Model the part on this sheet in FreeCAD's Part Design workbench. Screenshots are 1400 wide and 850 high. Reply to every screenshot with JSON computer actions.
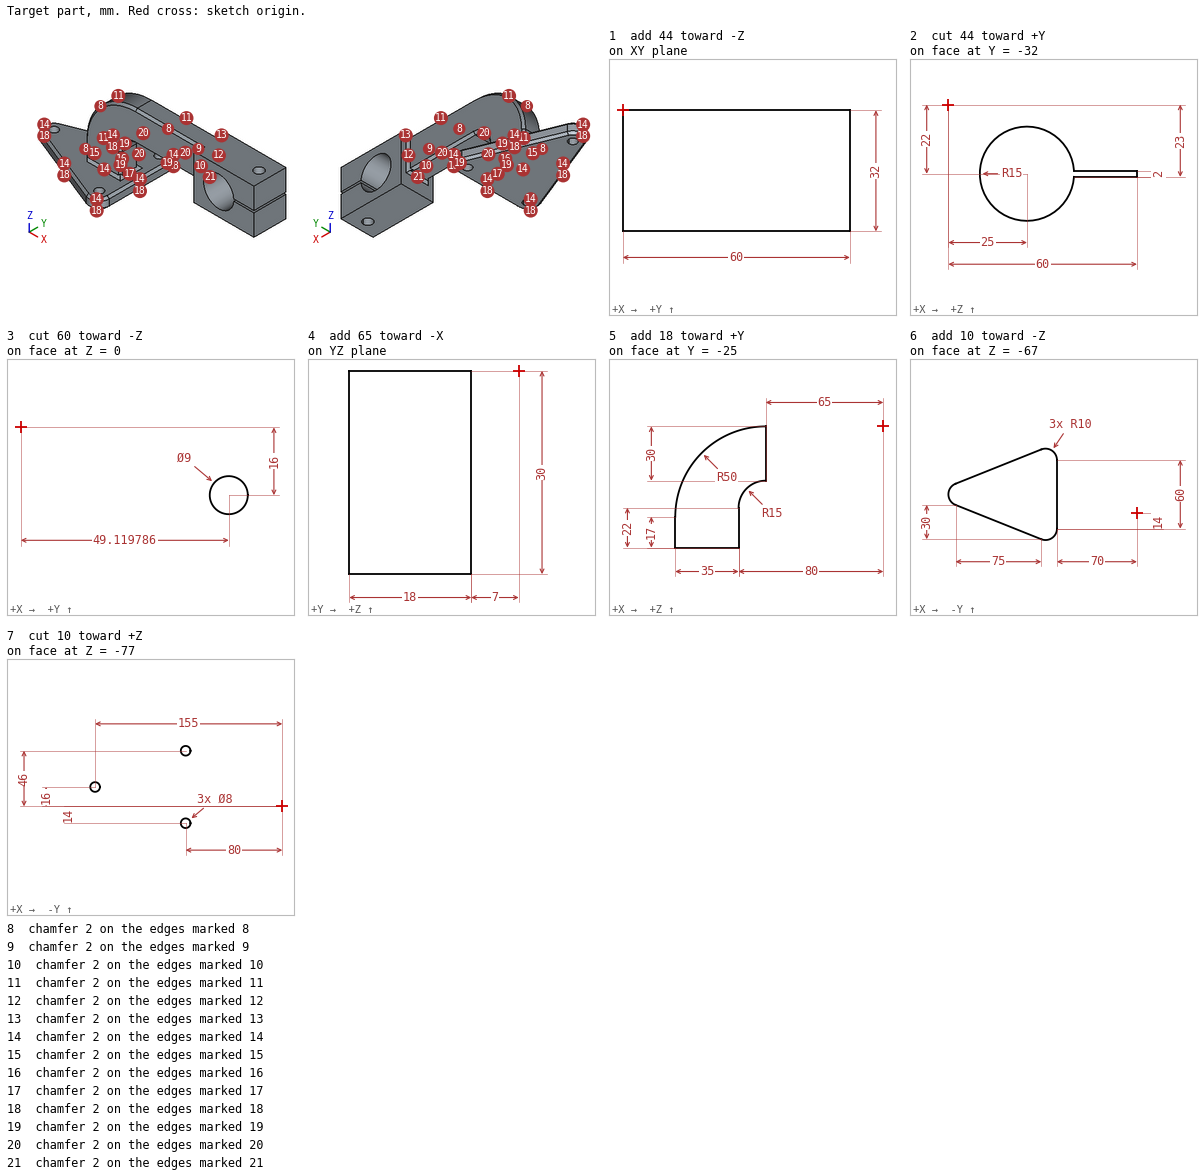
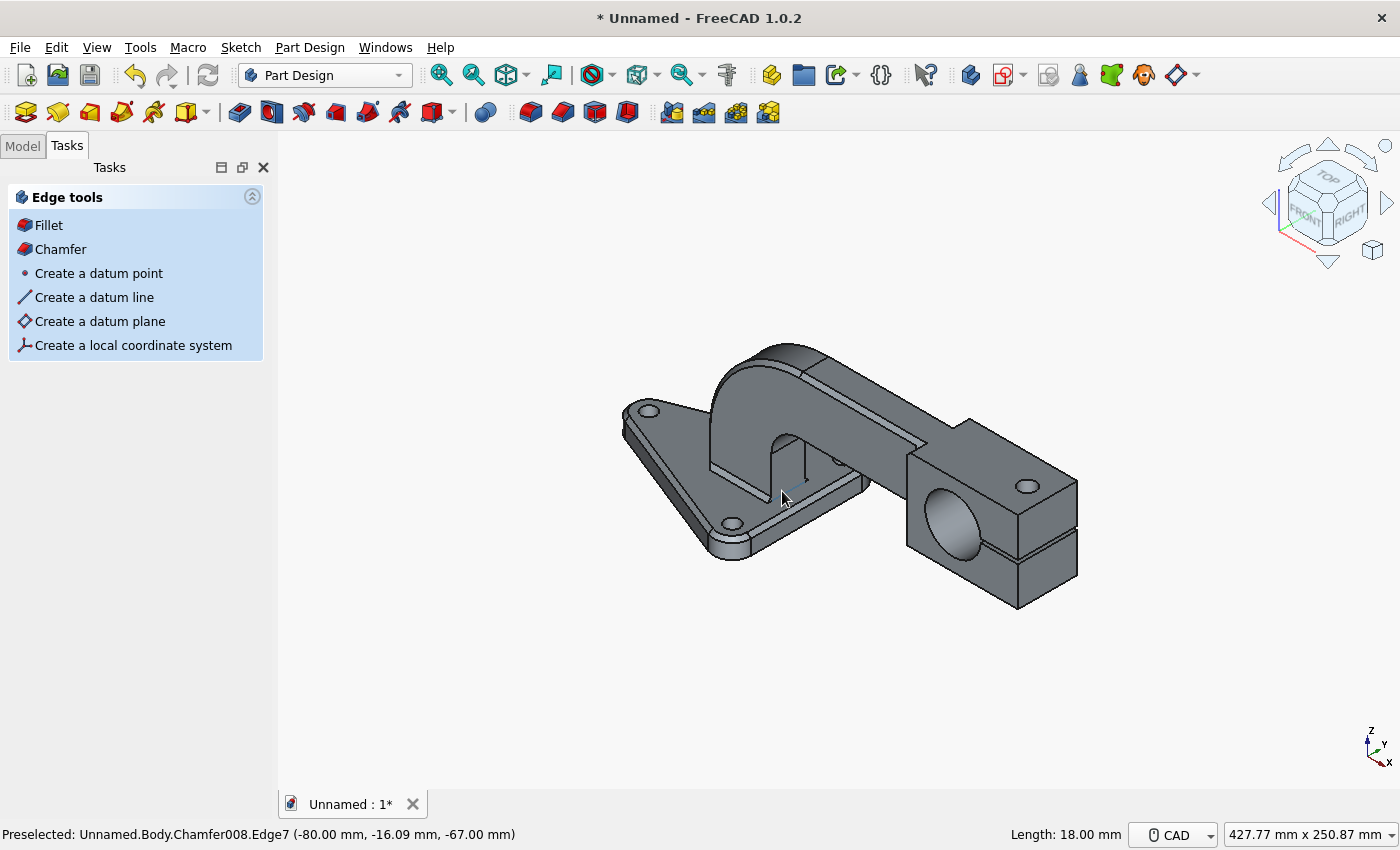
{"action": "left_click", "coordinate": [564, 112]}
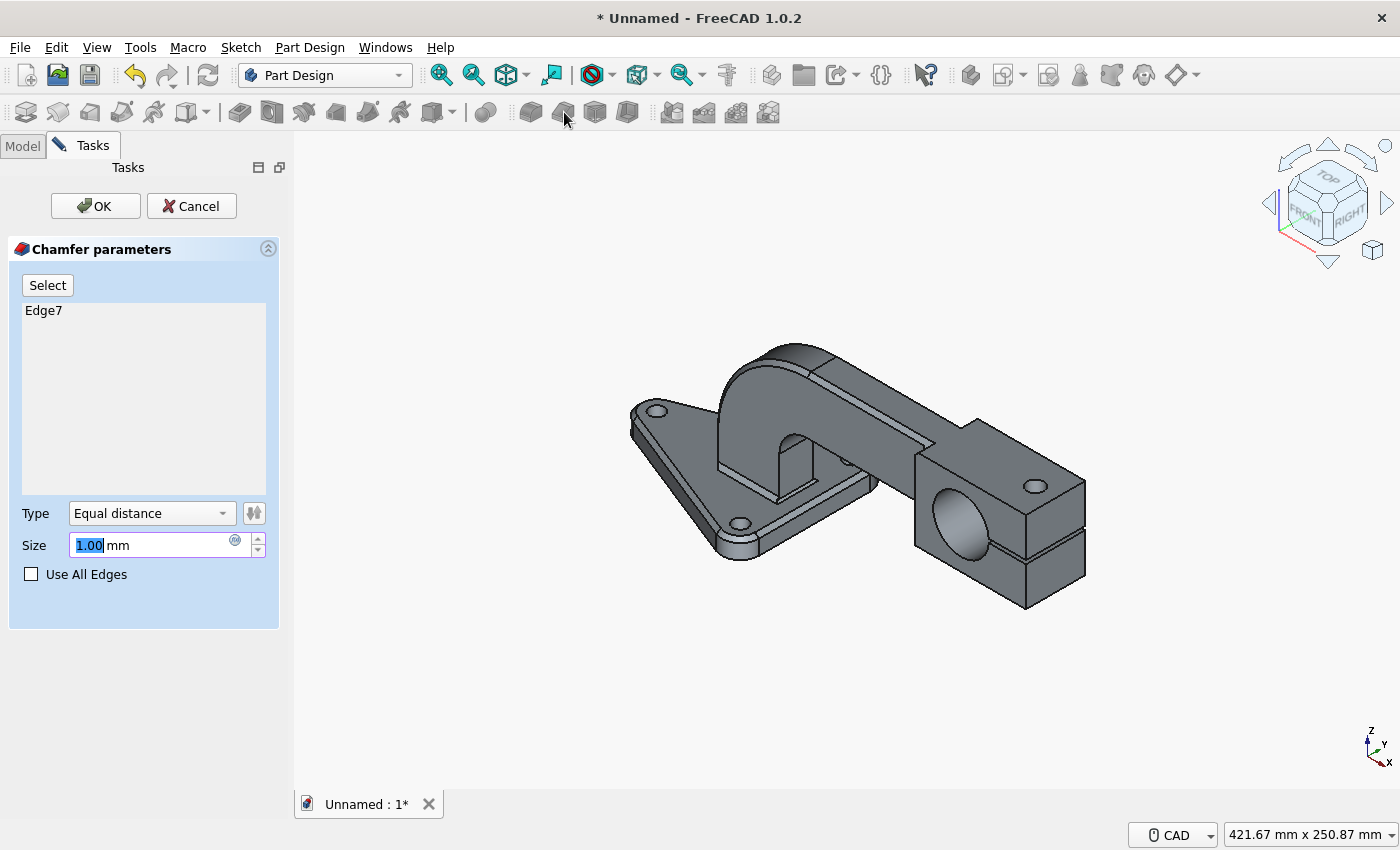
{"action": "type", "text": "2"}
{"action": "key", "text": "Tab"}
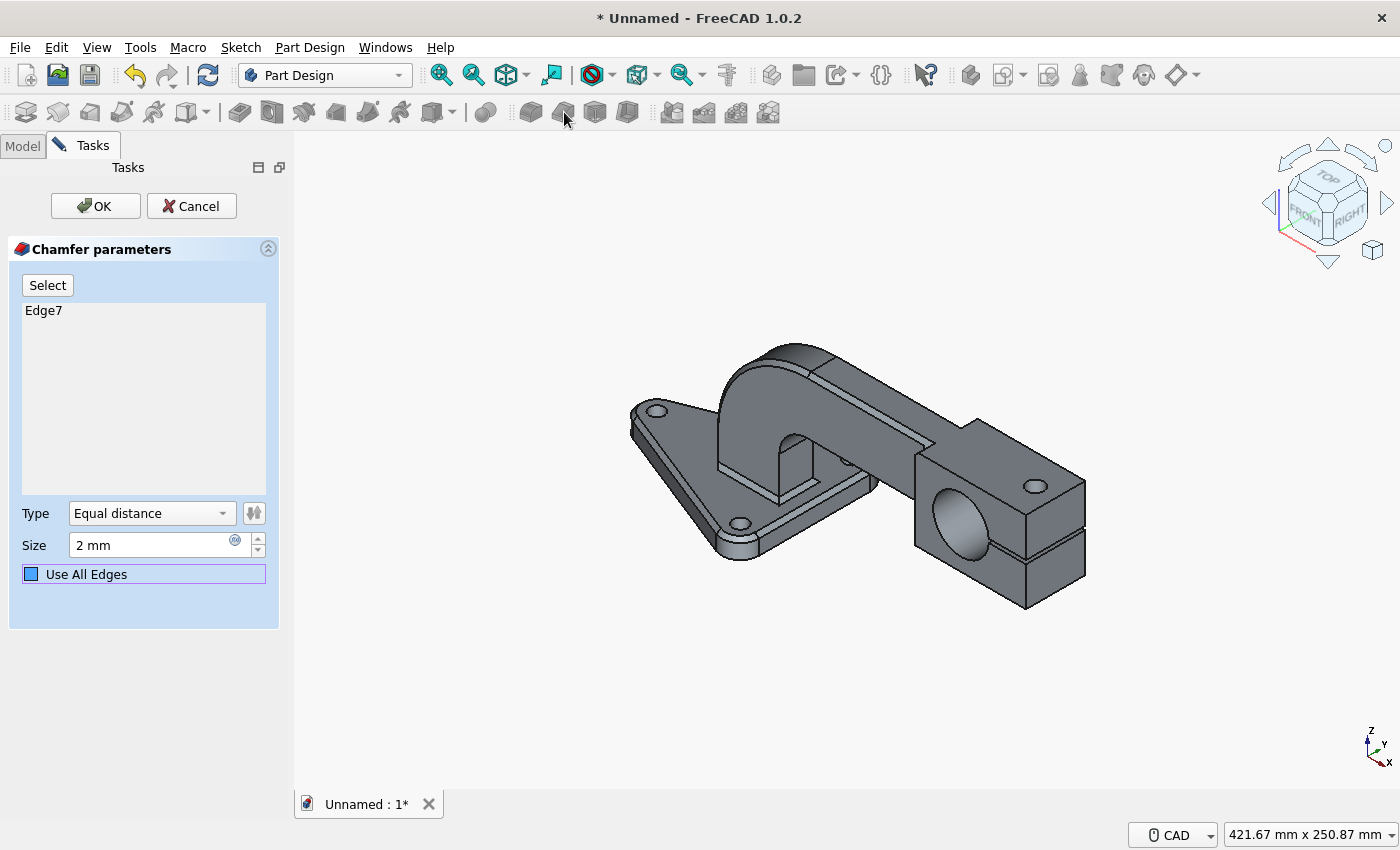
{"action": "left_click", "coordinate": [96, 206]}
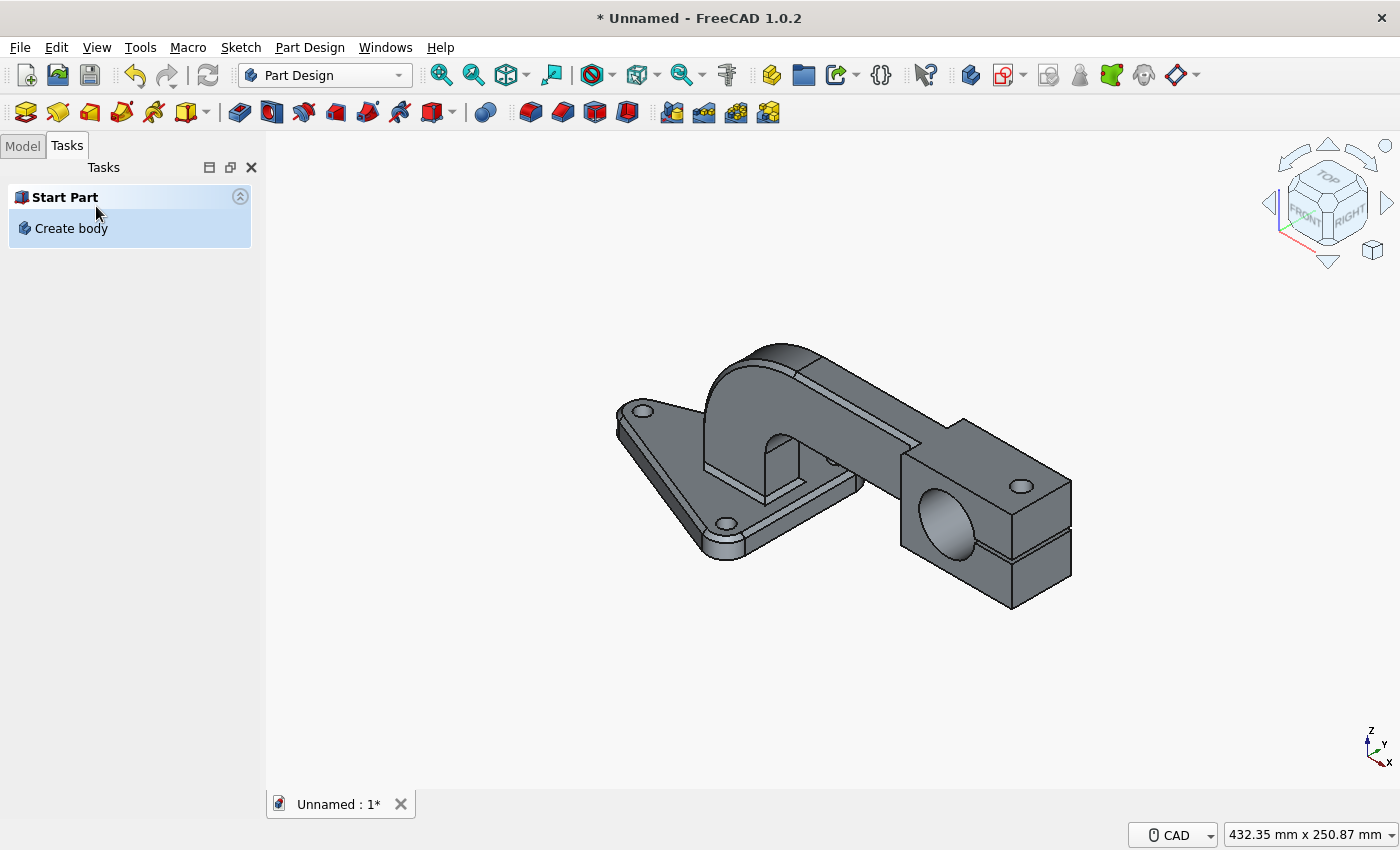
{"action": "left_click", "coordinate": [712, 557]}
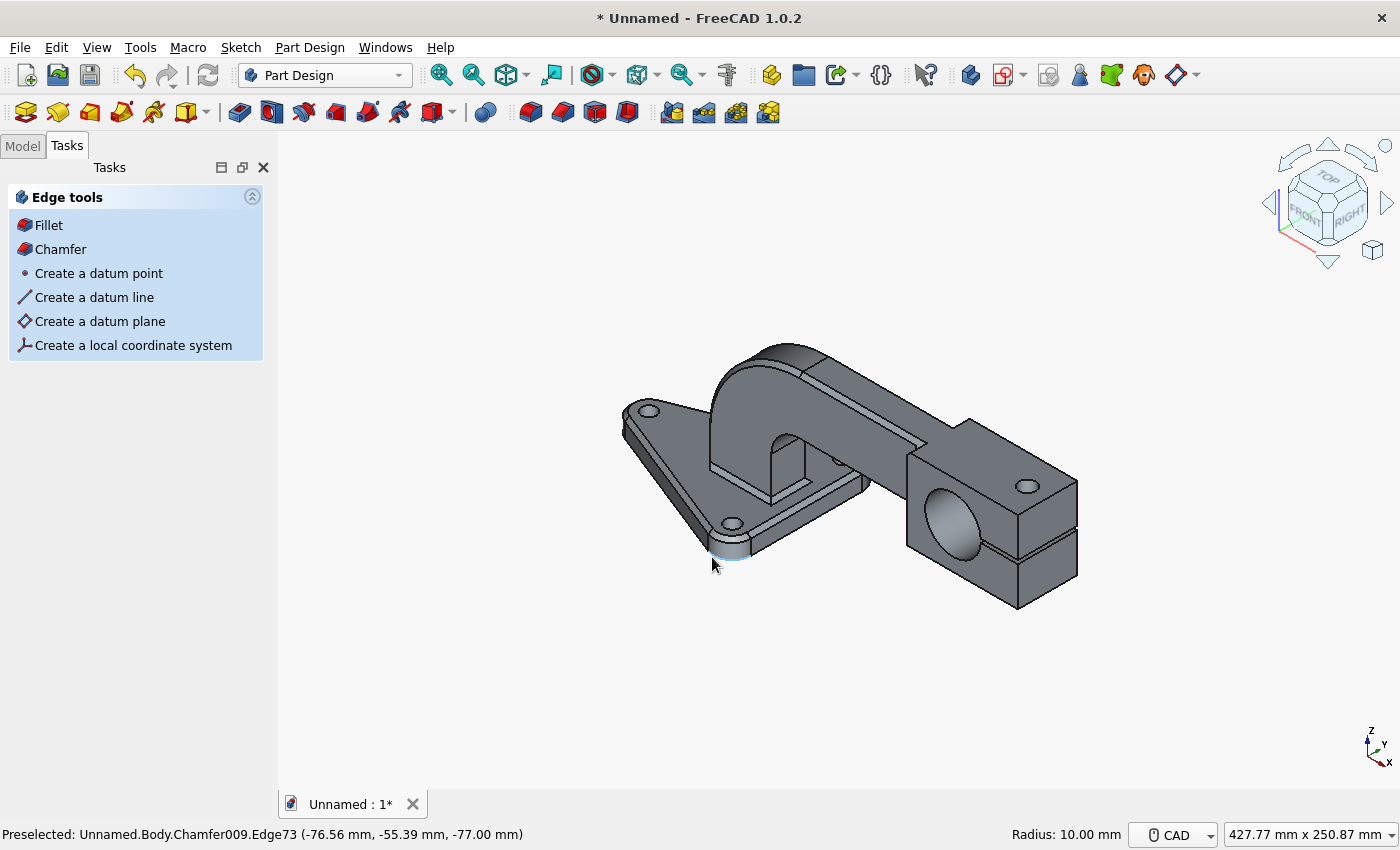
{"action": "key", "text": "2"}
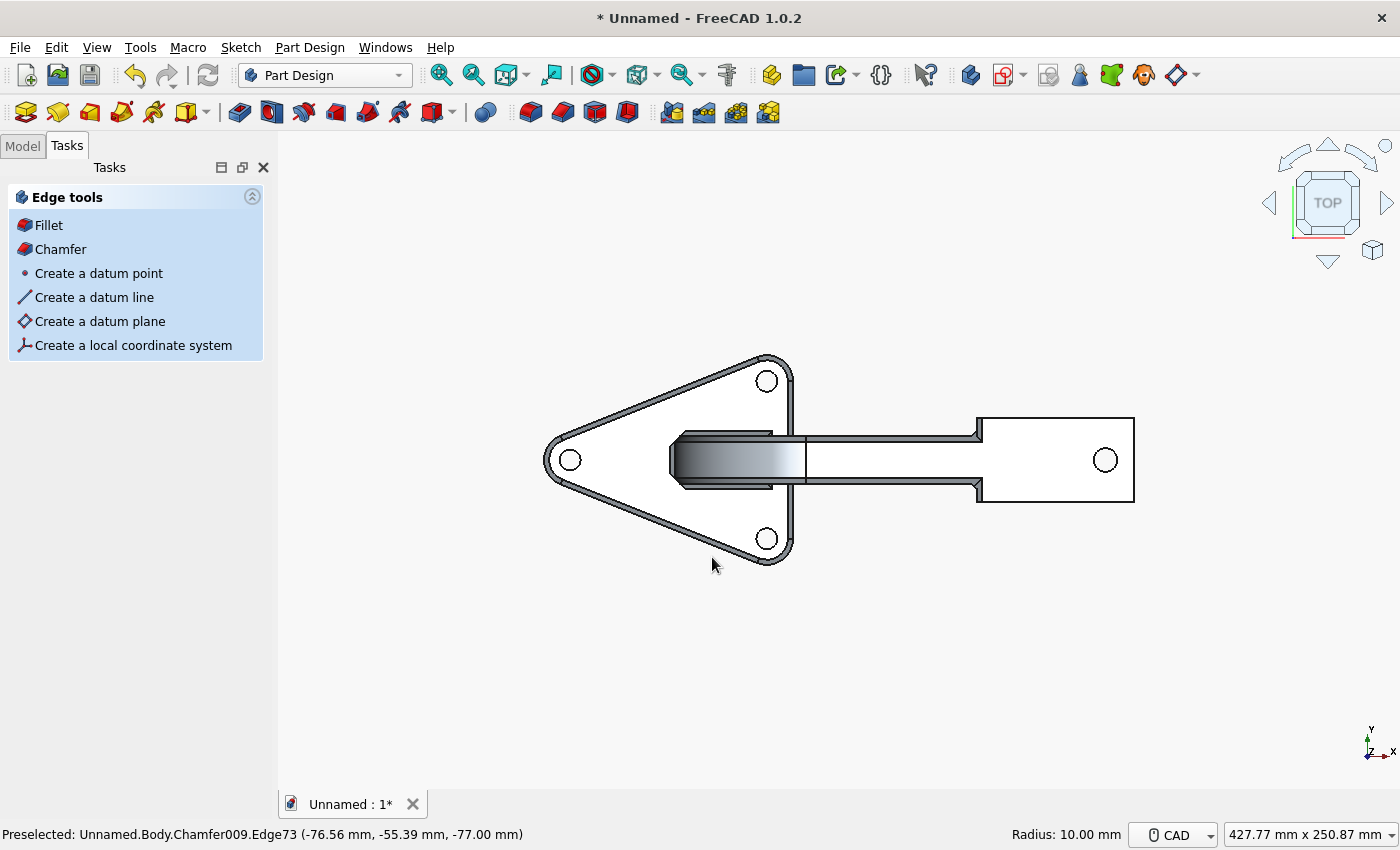
{"action": "key", "text": "0"}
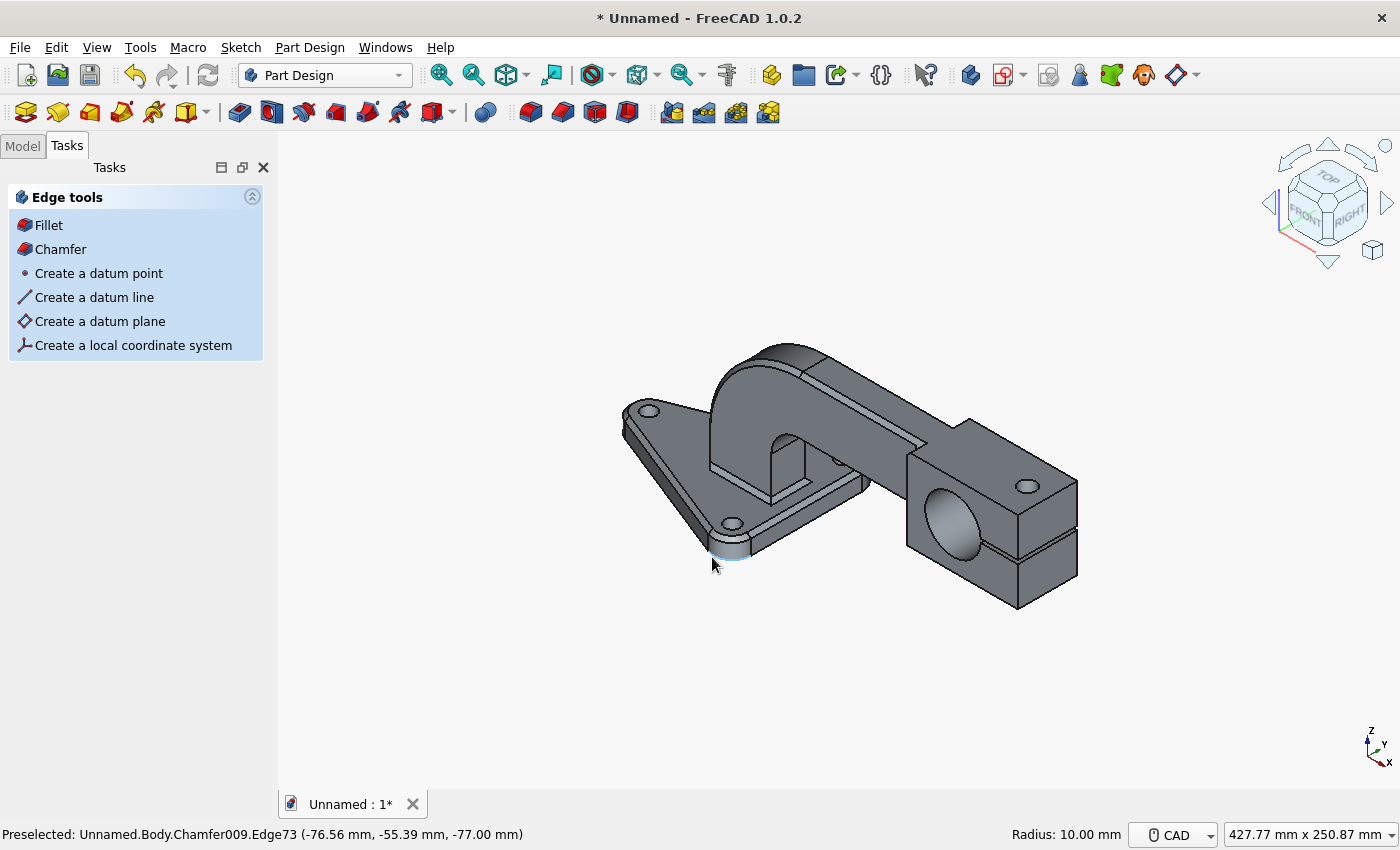
{"action": "key", "text": "1"}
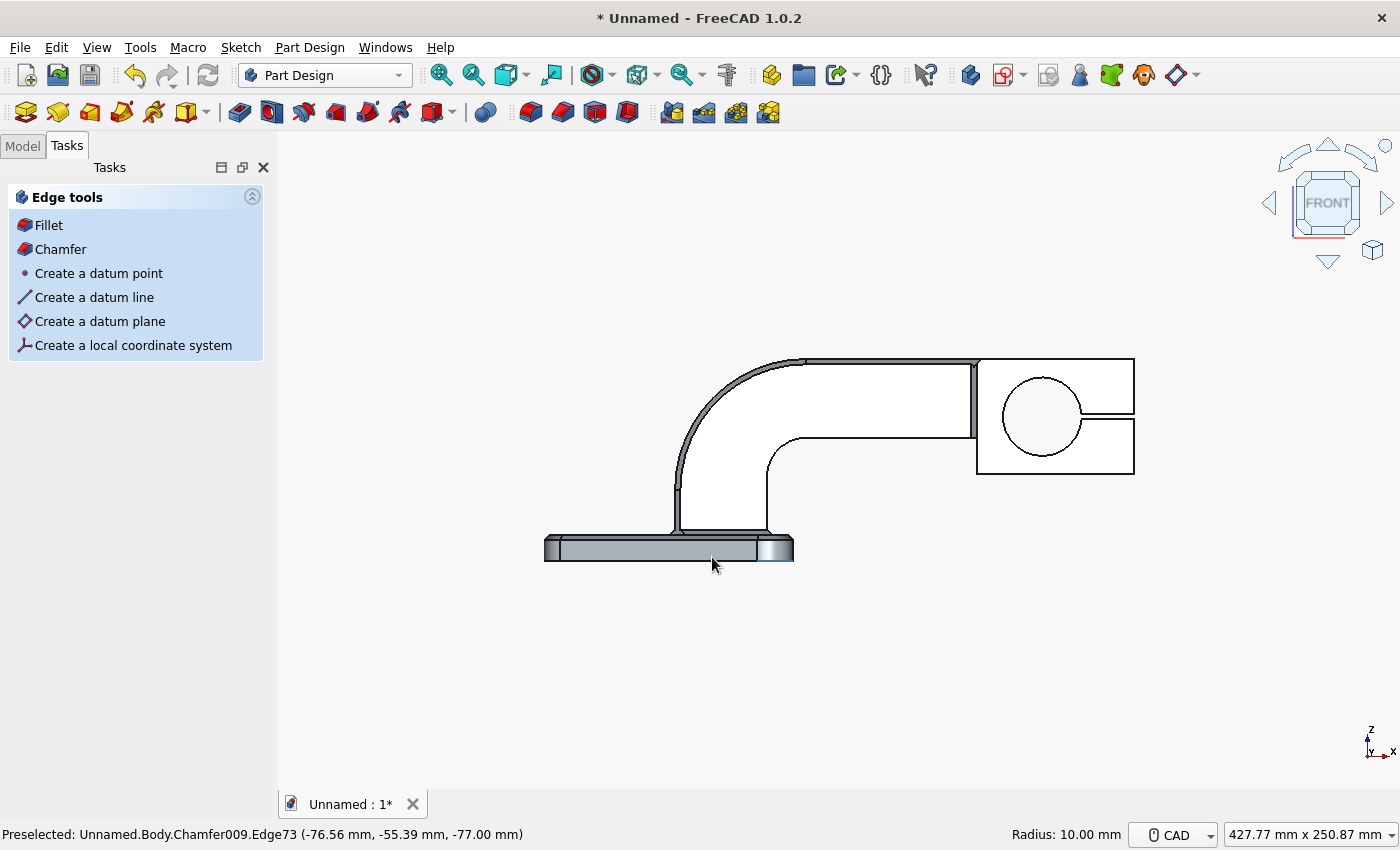
{"action": "left_click", "coordinate": [659, 560], "text": "ctrl"}